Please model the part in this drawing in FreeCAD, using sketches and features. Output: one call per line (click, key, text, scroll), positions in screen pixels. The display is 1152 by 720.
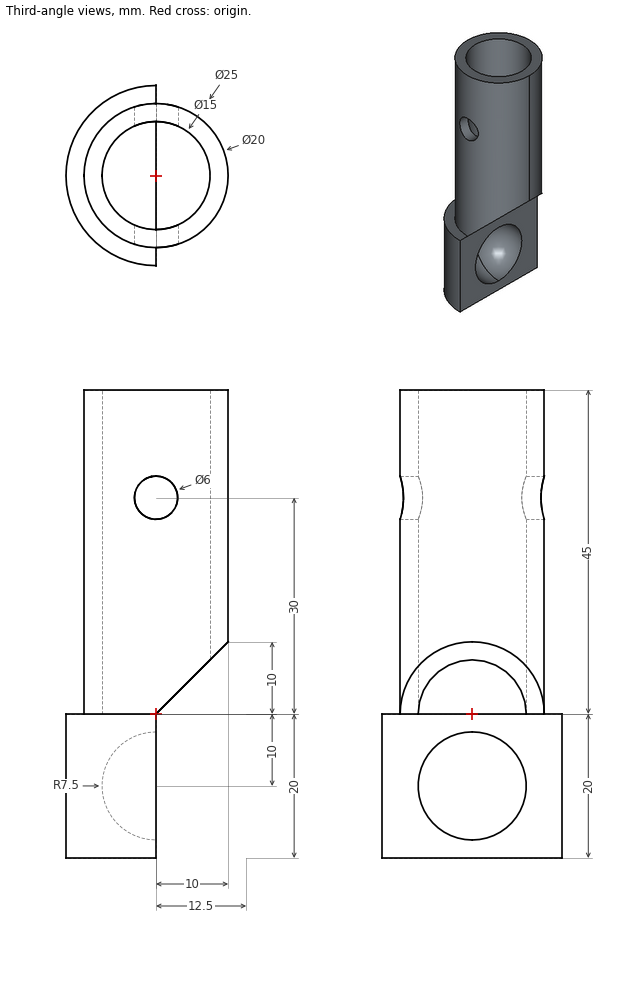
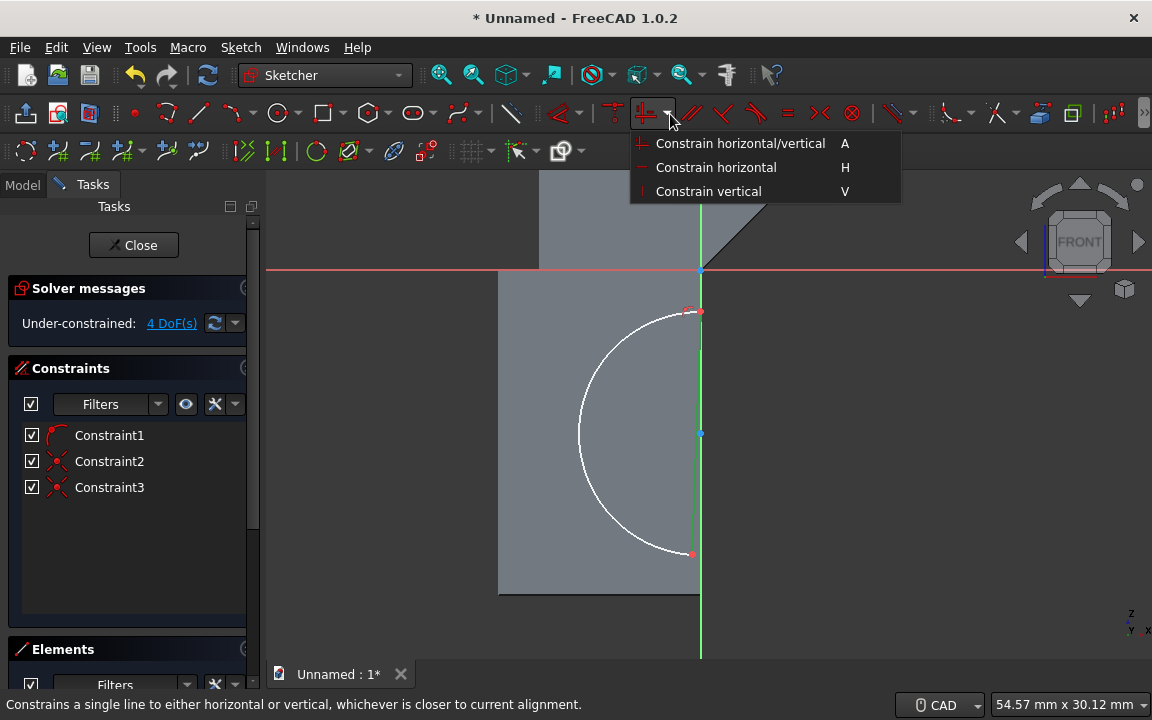
click(766, 191)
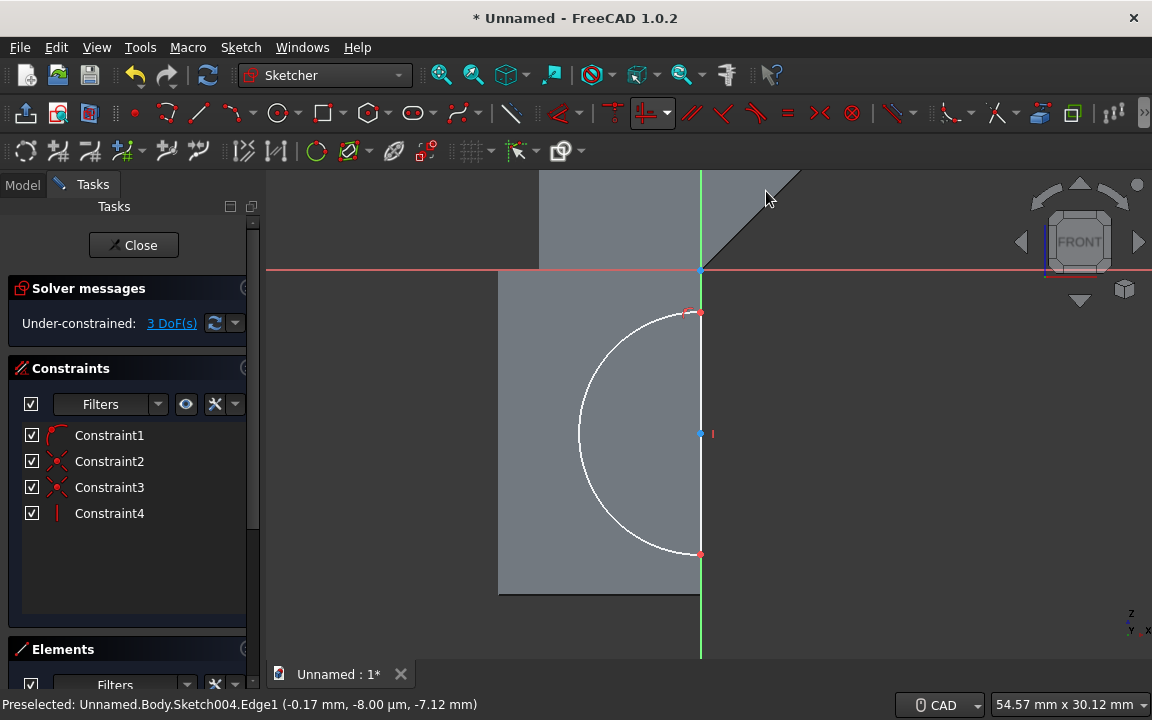
click(701, 434)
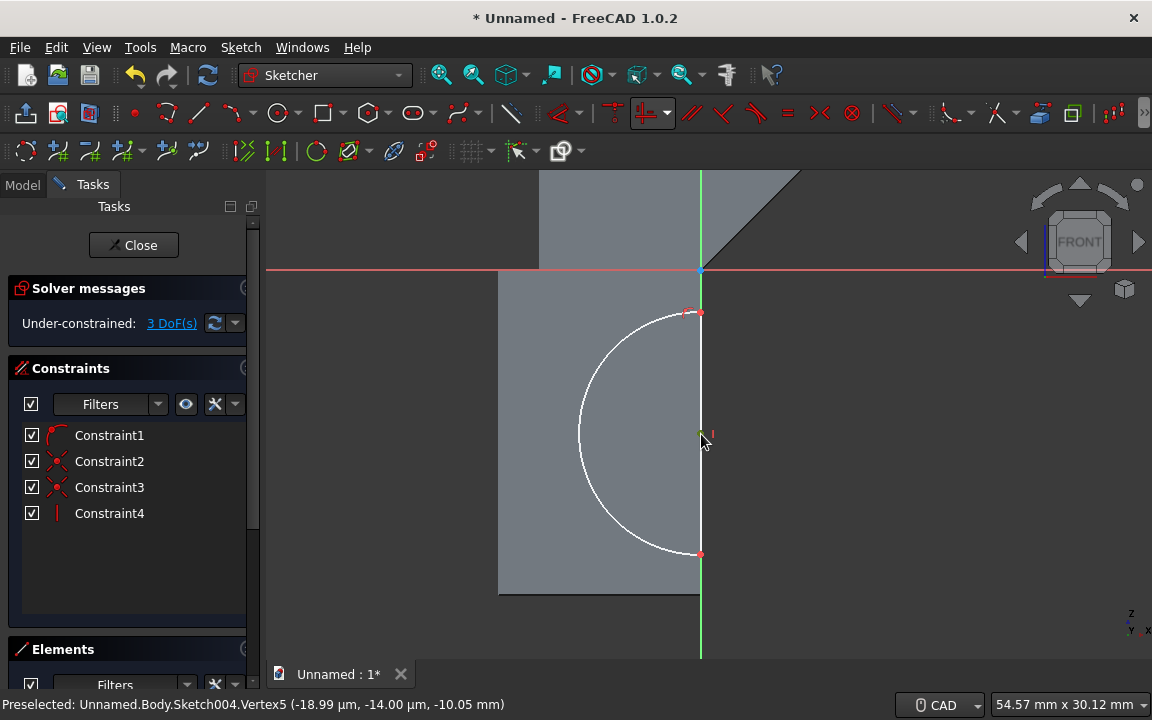
click(701, 600)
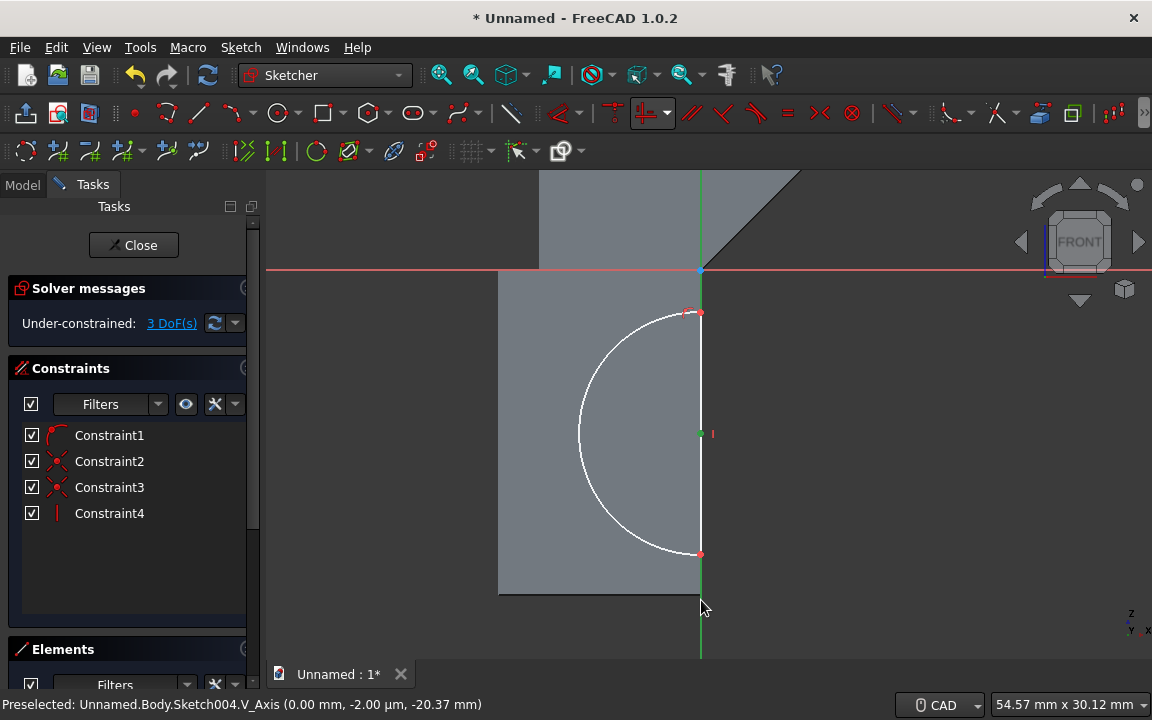
click(614, 114)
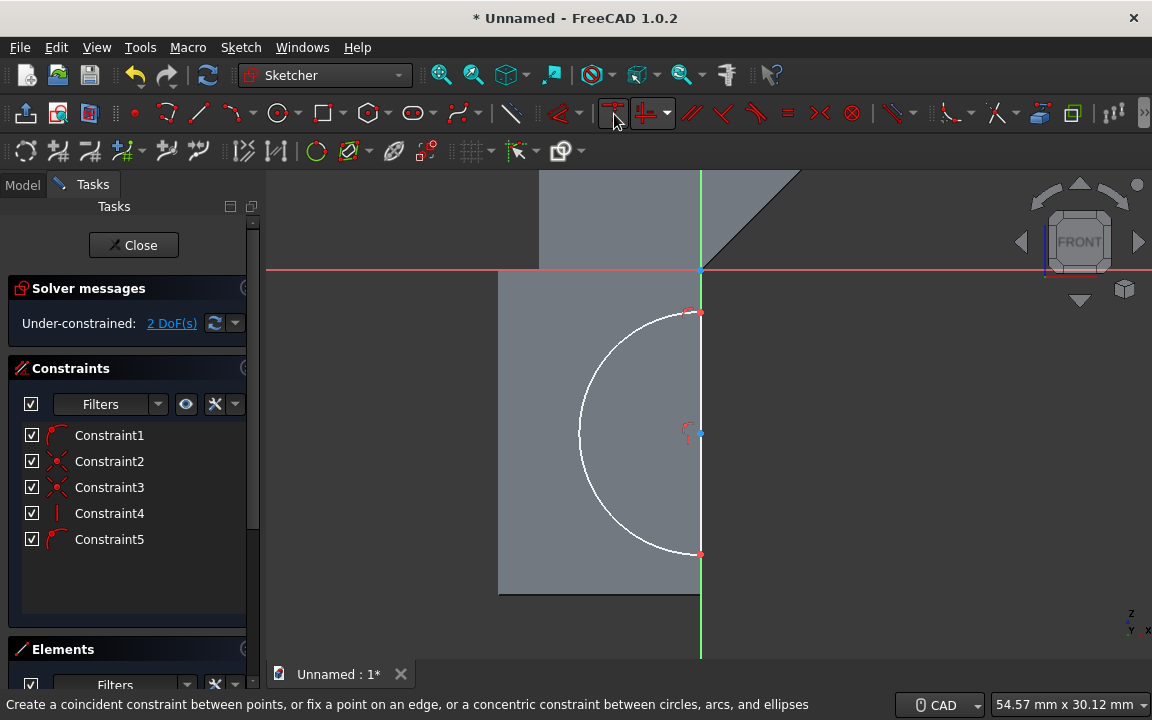
click(558, 114)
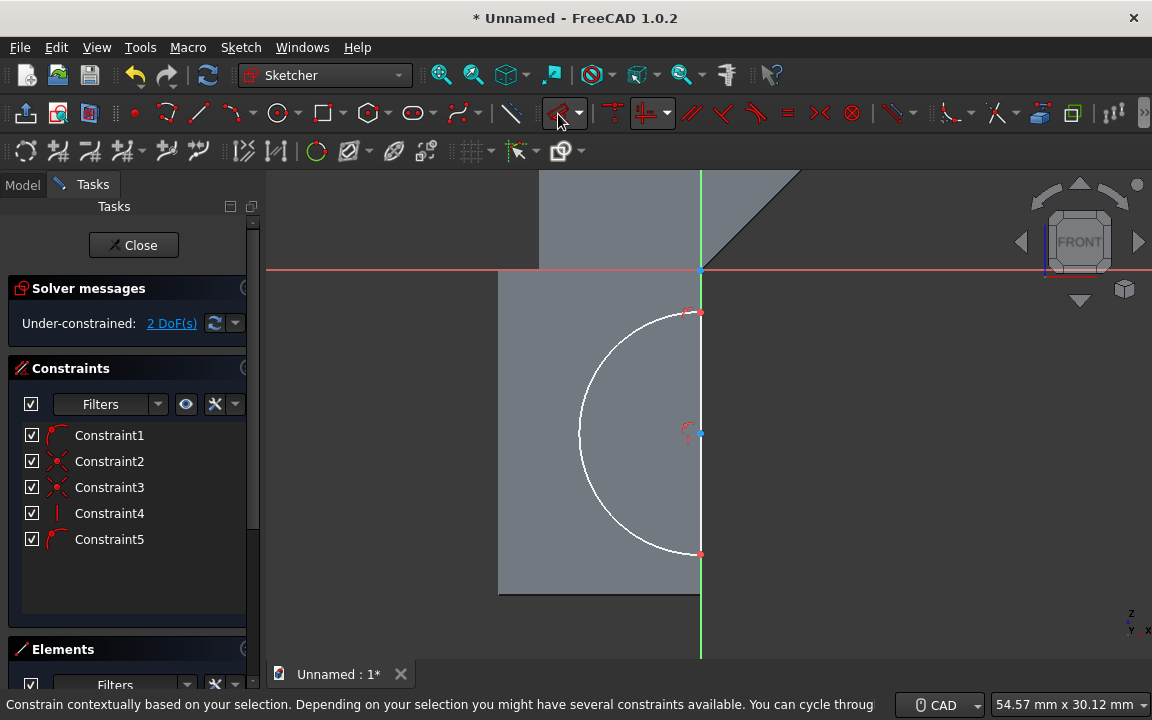
click(603, 362)
click(577, 343)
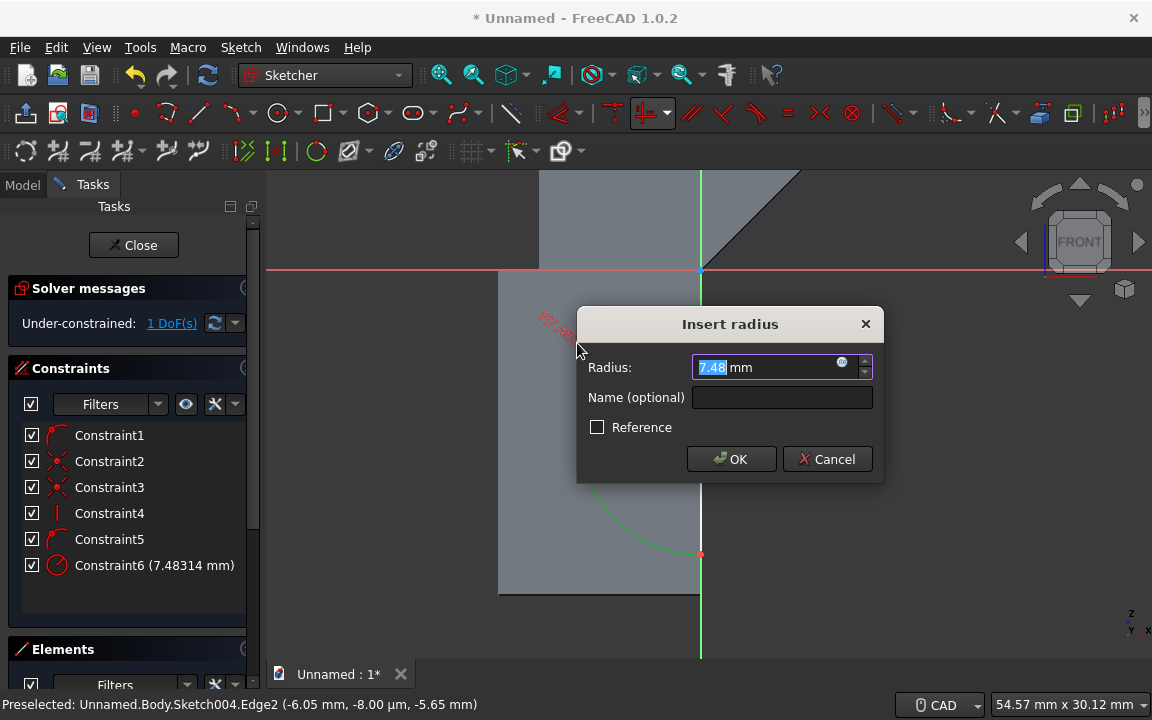
text(7.5)
key(Return)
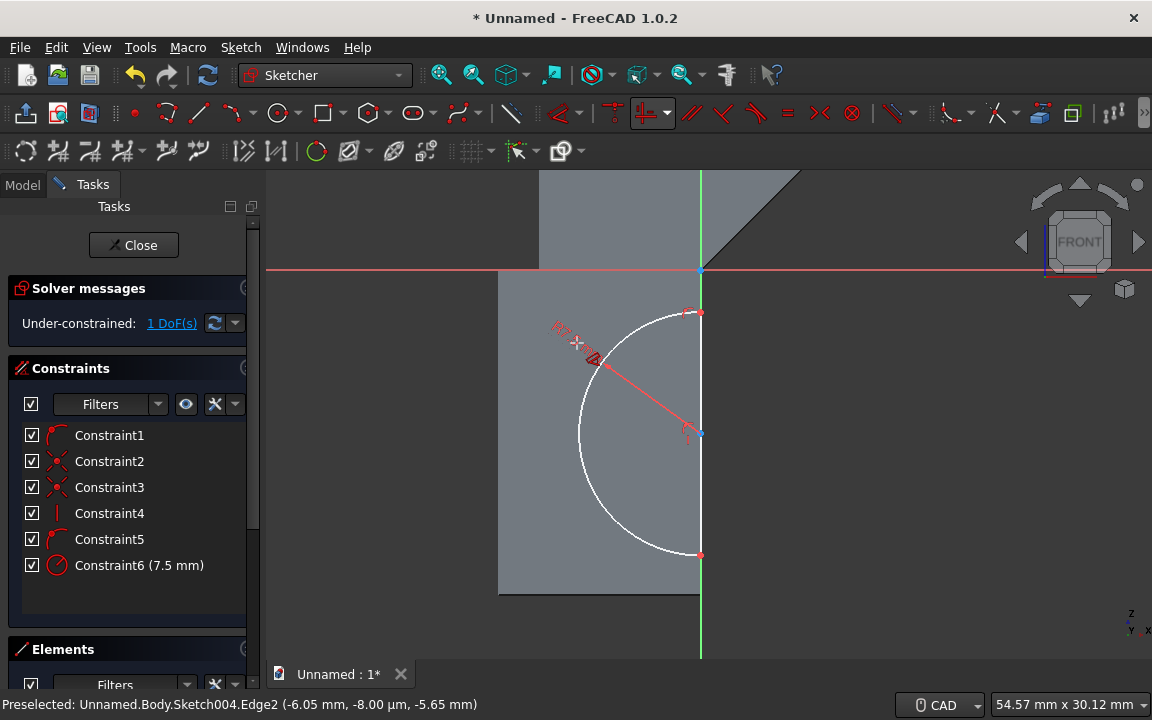
click(701, 434)
click(735, 352)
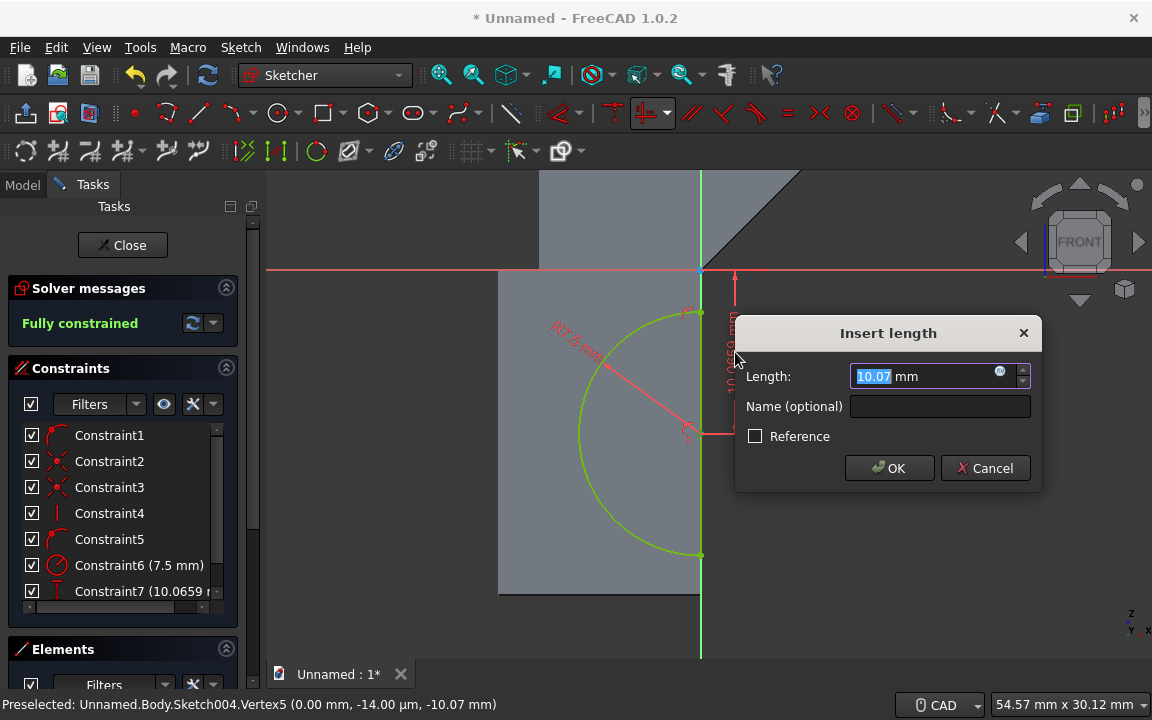
text(10)
key(Return)
key(Escape)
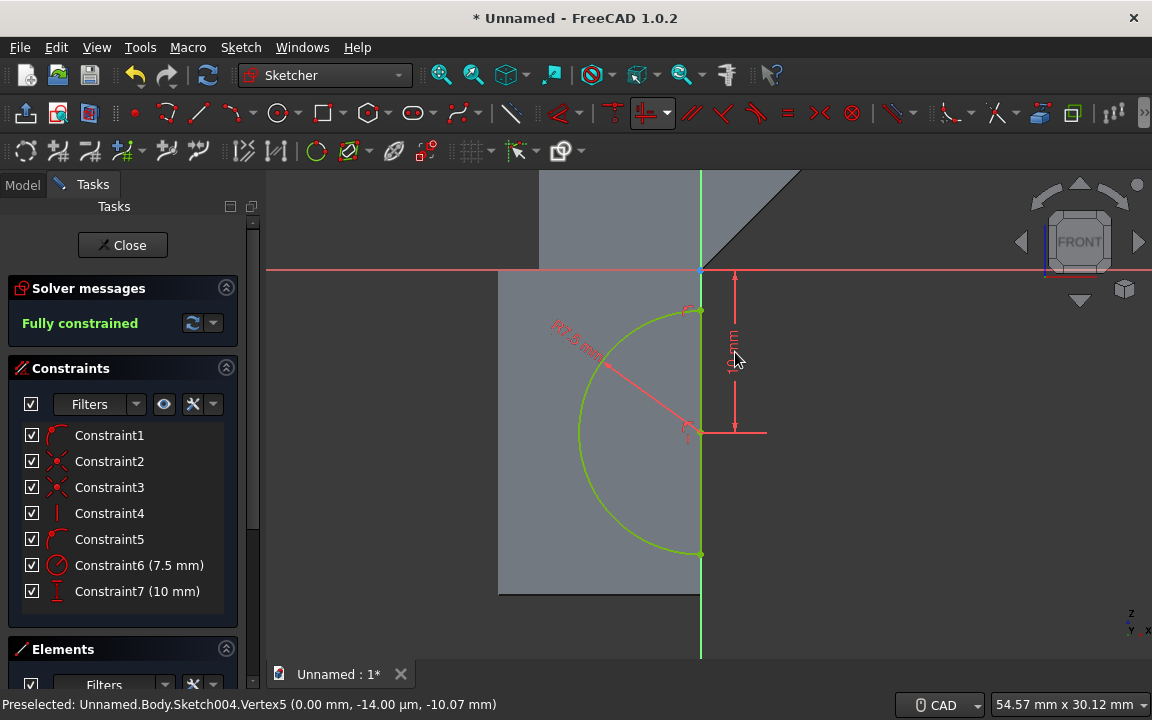
click(123, 245)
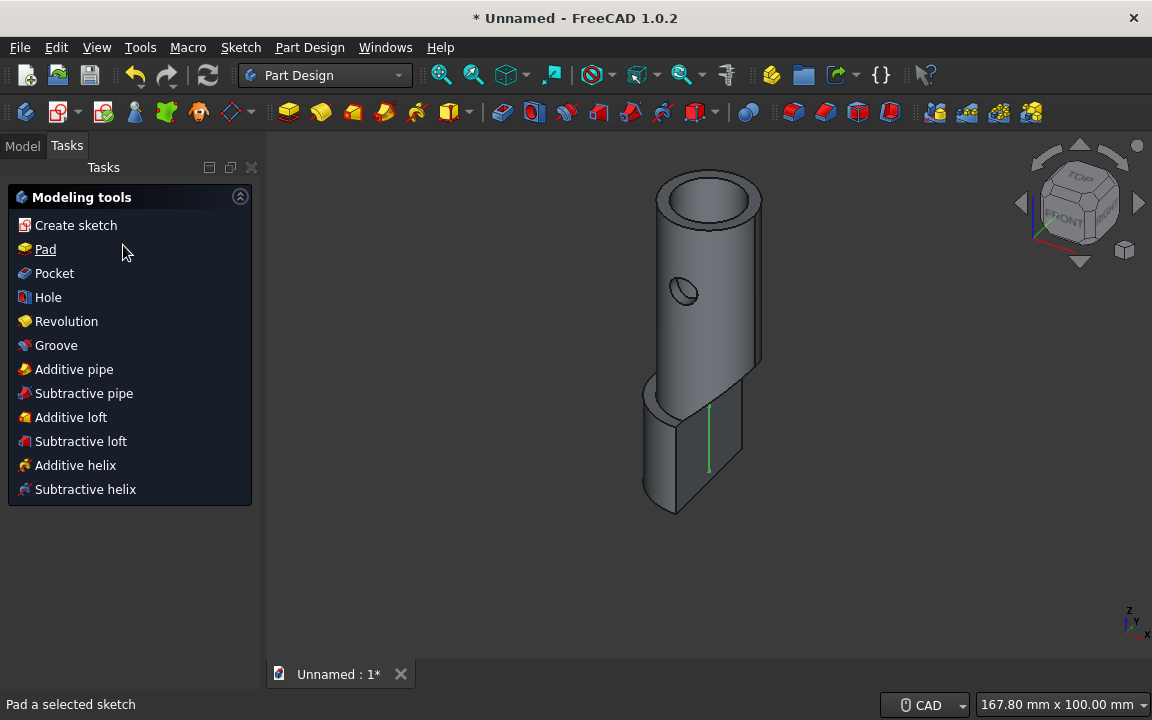
click(568, 112)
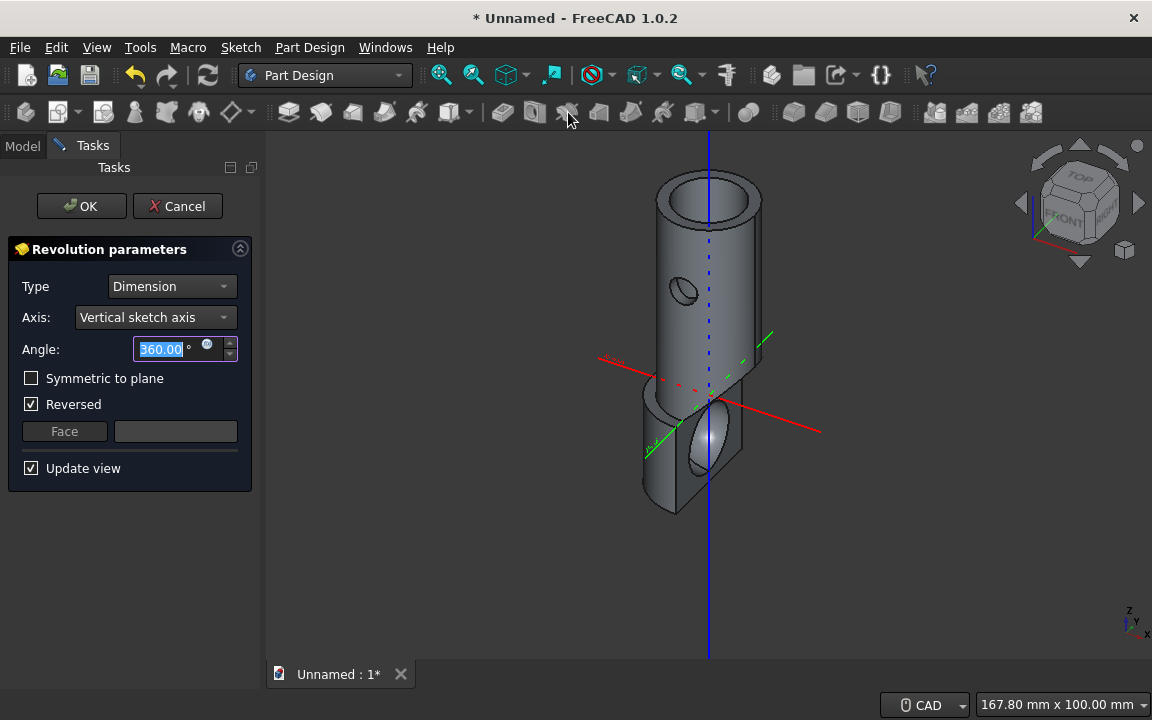
click(82, 206)